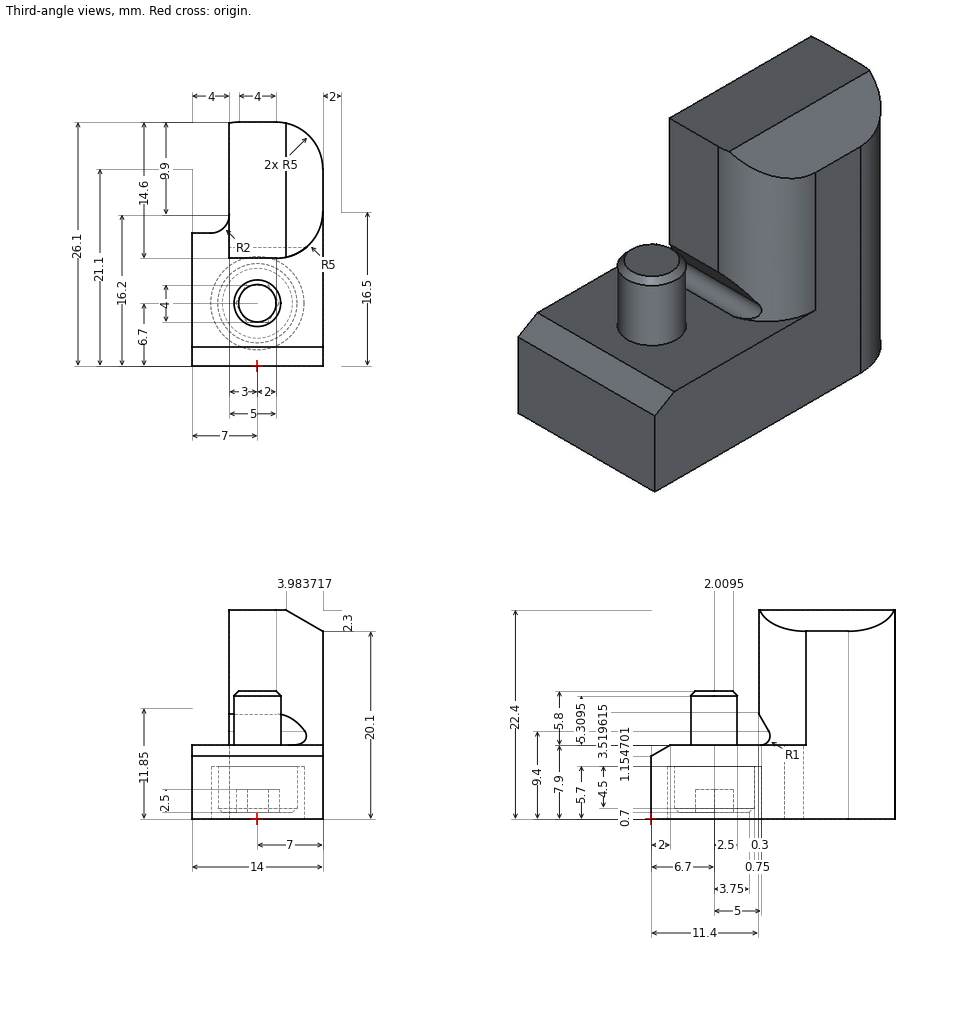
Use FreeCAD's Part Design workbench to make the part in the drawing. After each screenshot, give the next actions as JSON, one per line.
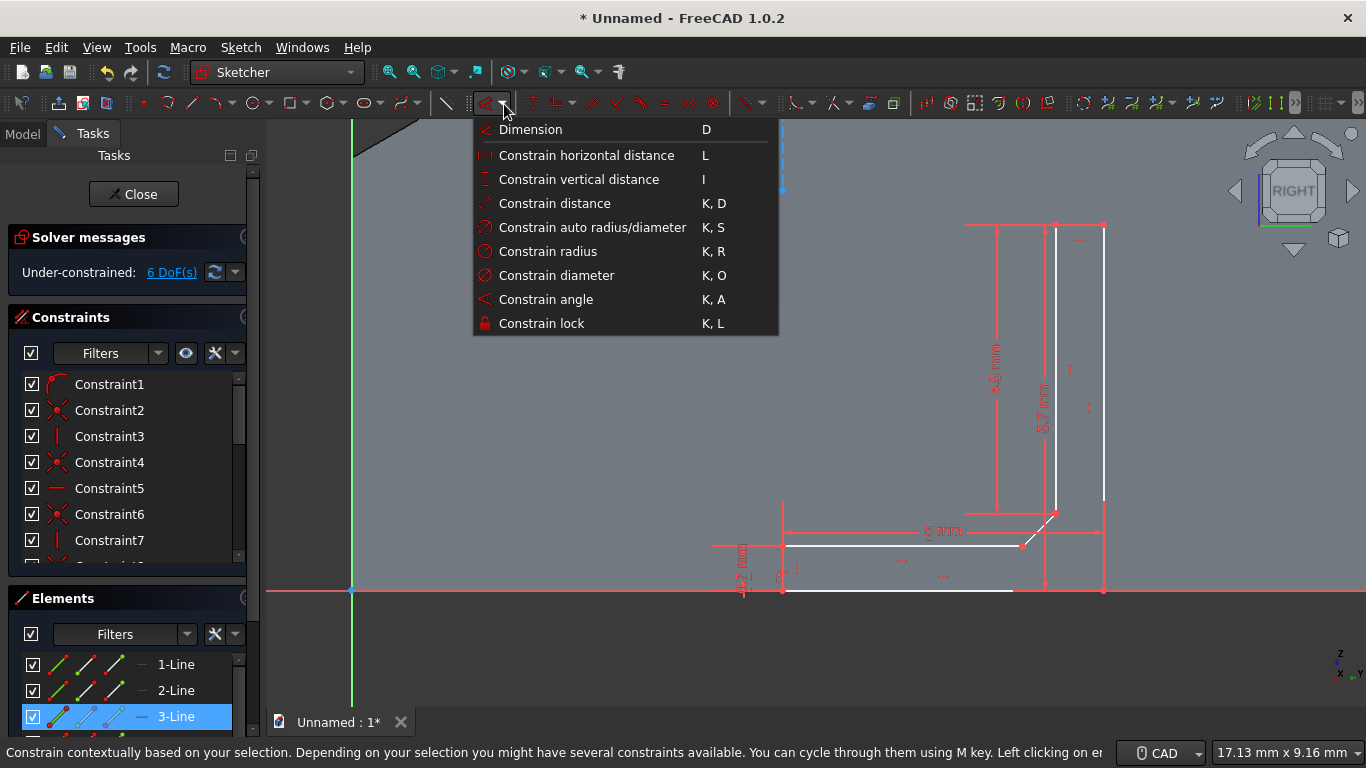
{"action": "left_click", "coordinate": [626, 155]}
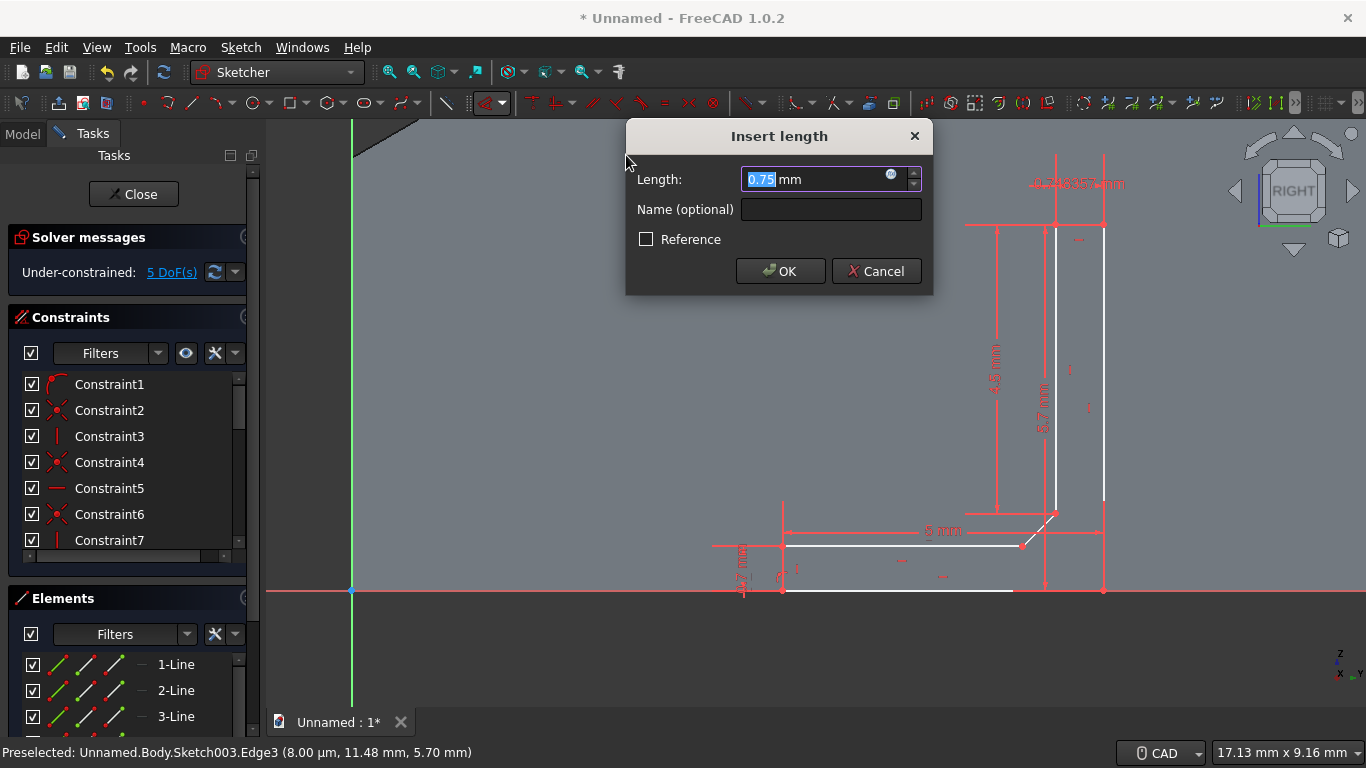
{"action": "type", "text": "0.75"}
{"action": "key", "text": "Return"}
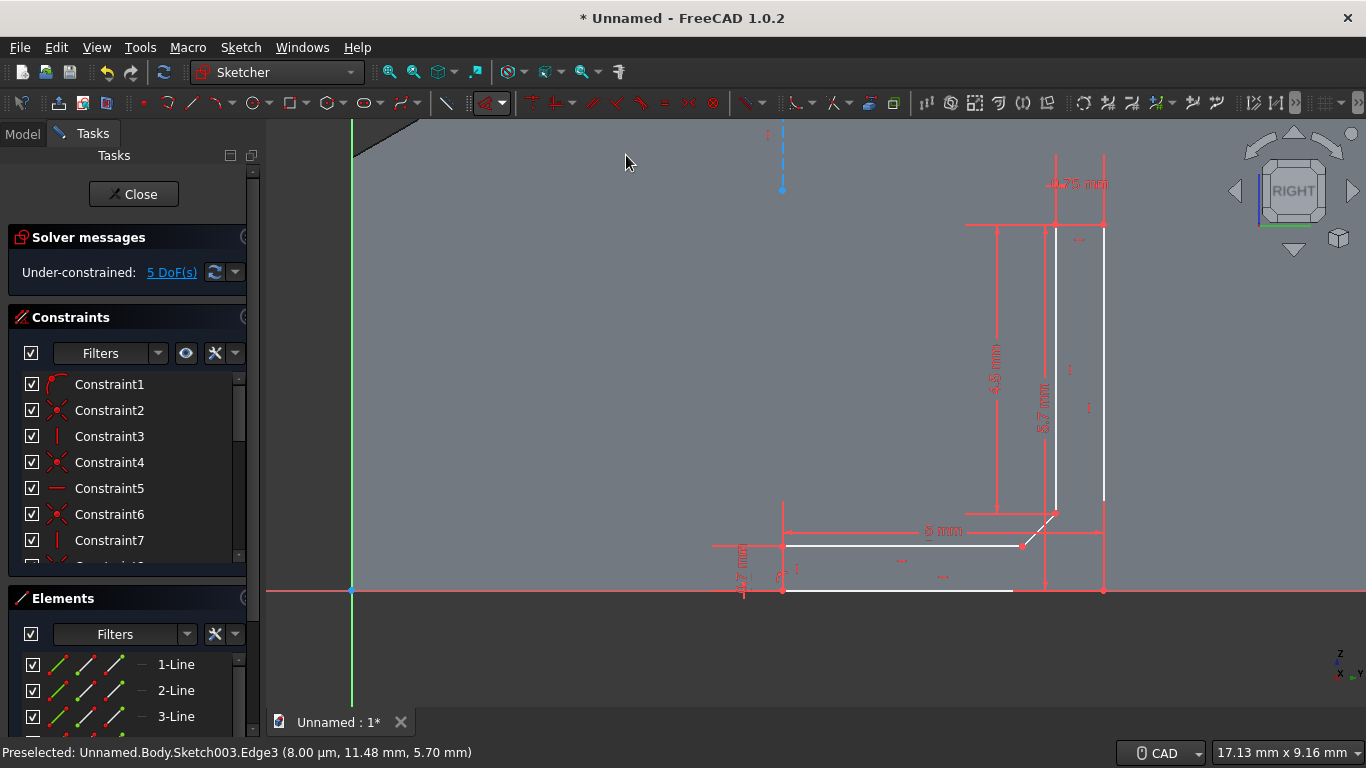
{"action": "left_click", "coordinate": [951, 546]}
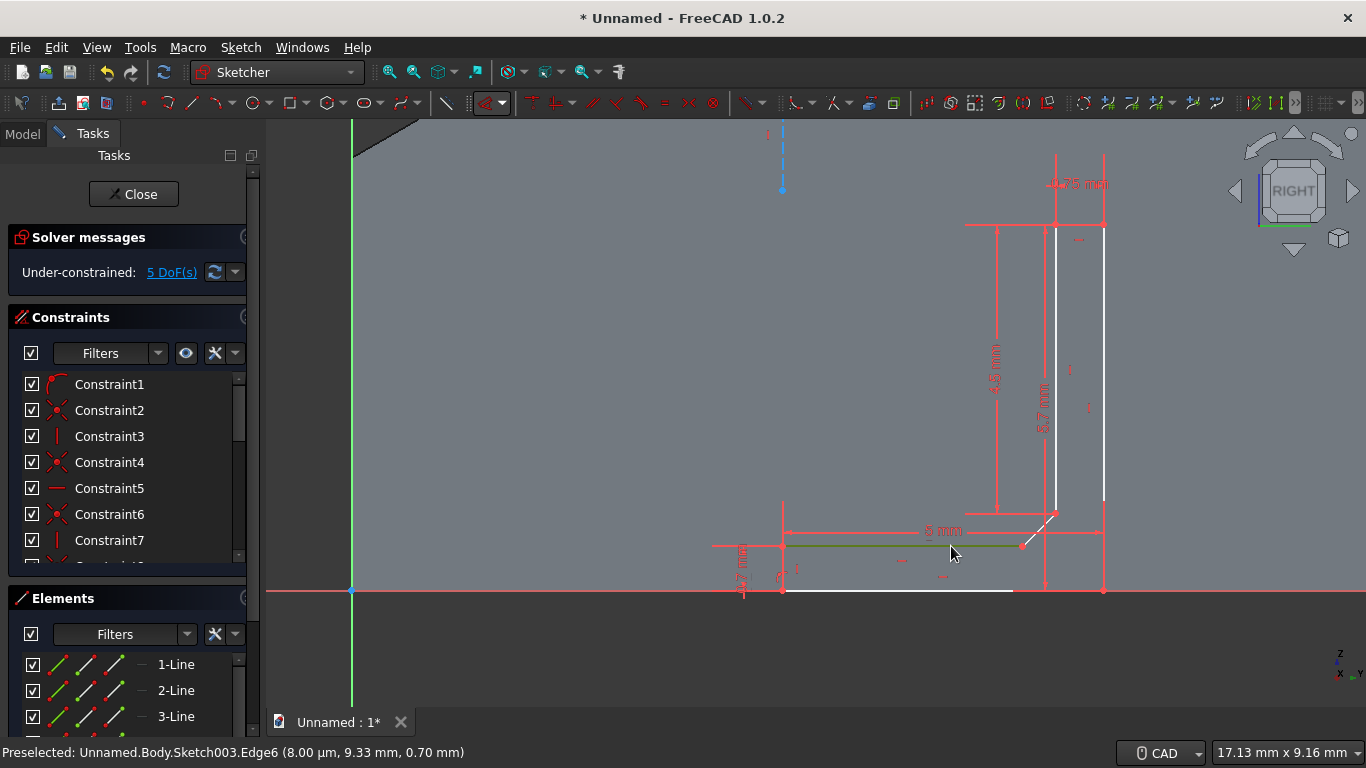
{"action": "key", "text": "l"}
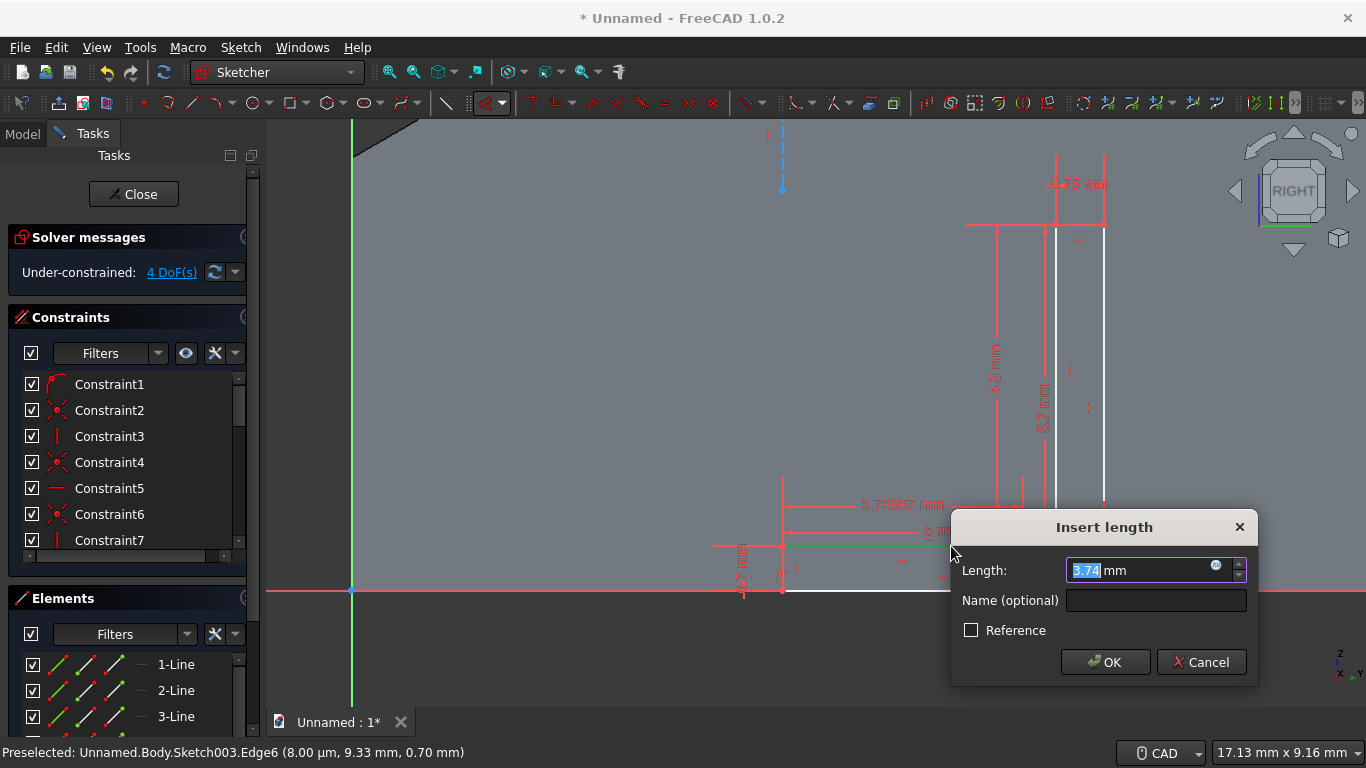
{"action": "type", "text": "3.75"}
{"action": "key", "text": "Return"}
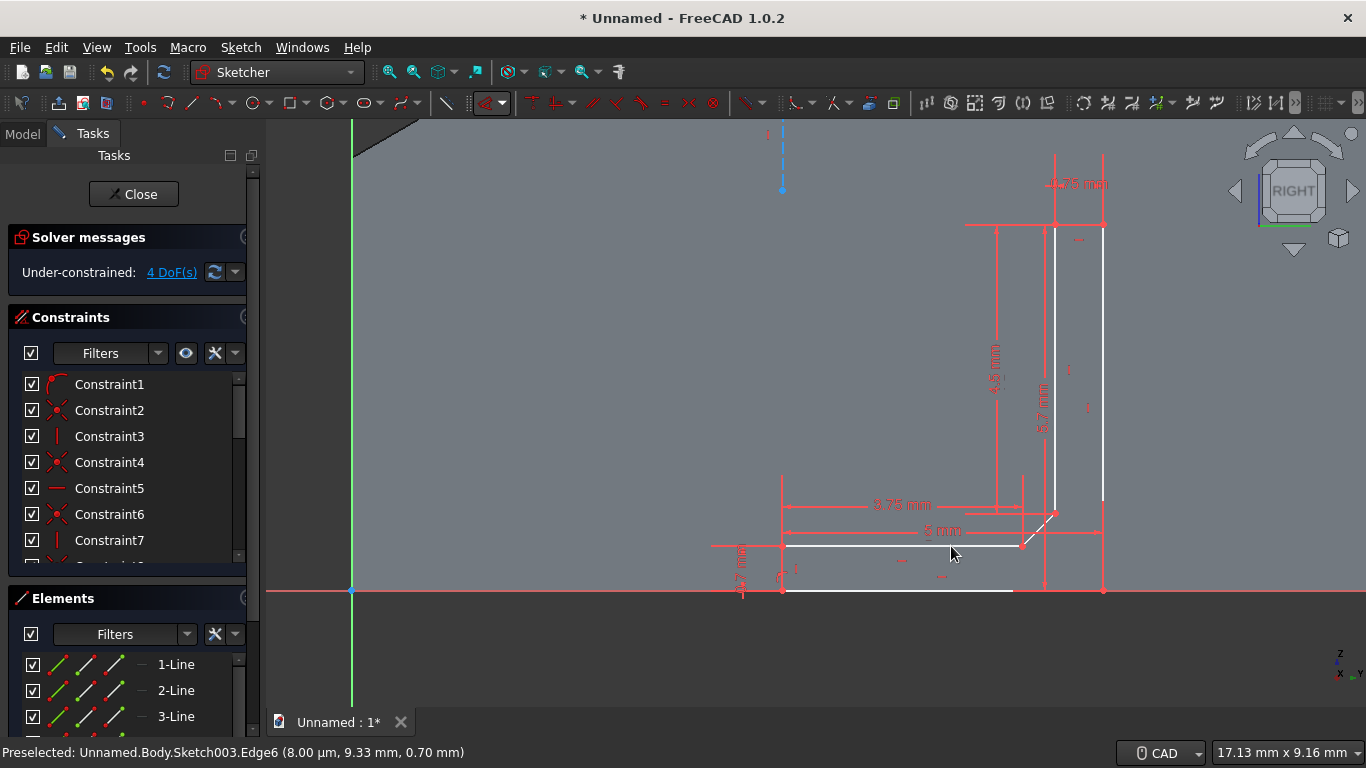
{"action": "left_click", "coordinate": [782, 591]}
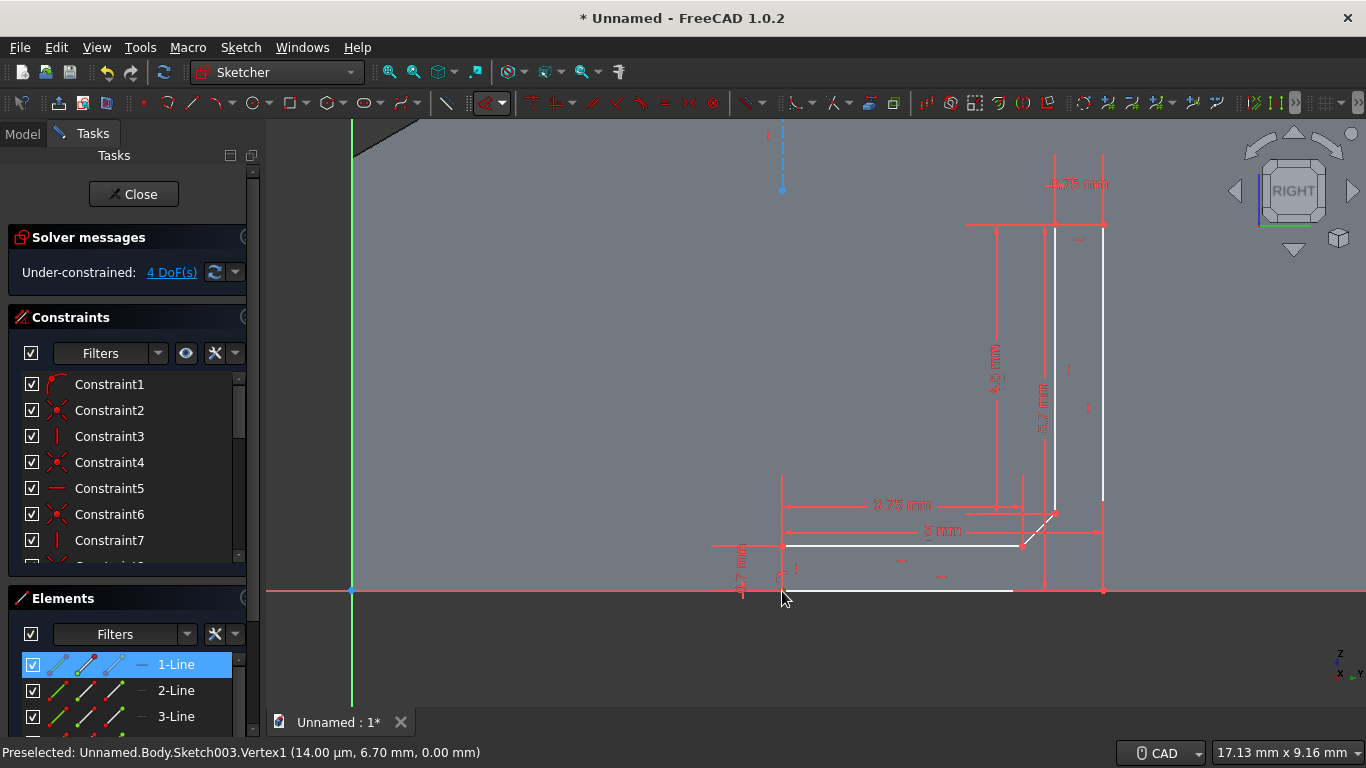
{"action": "left_click", "coordinate": [504, 104]}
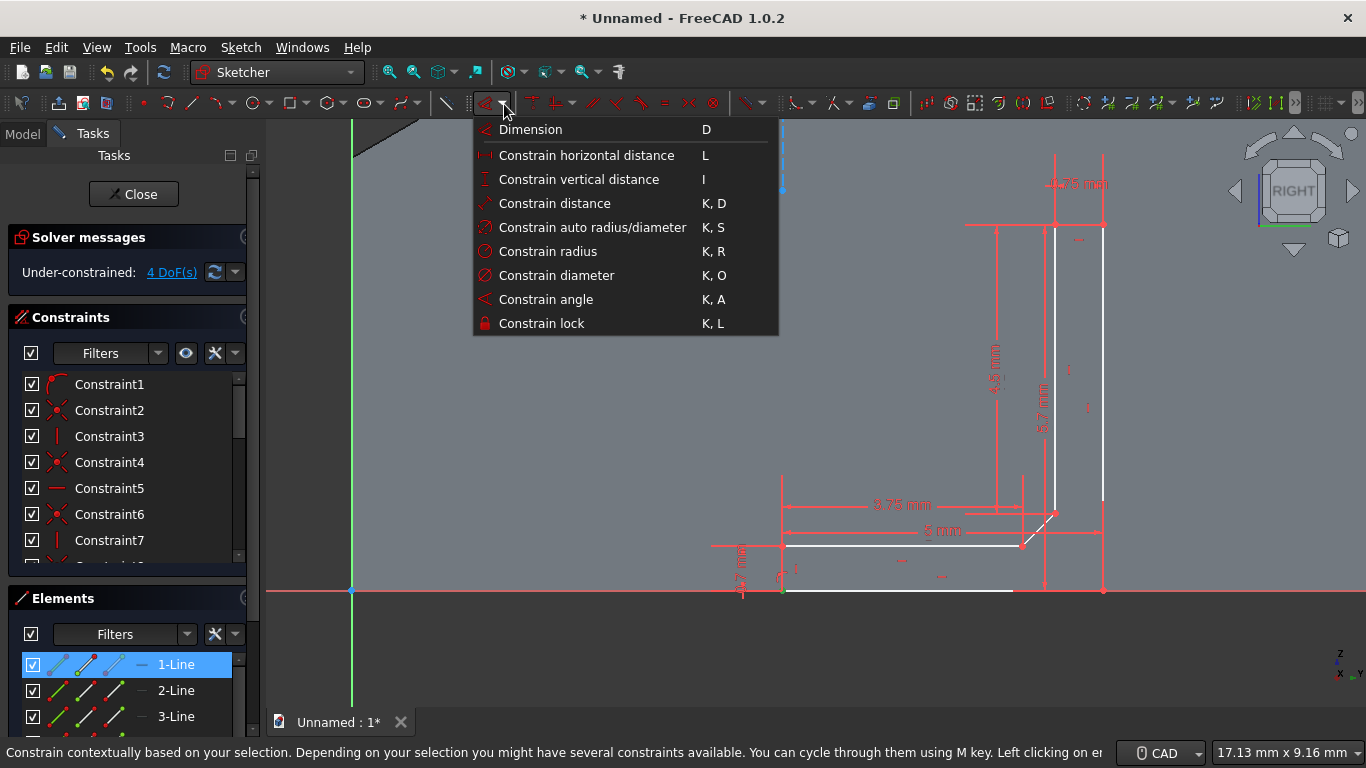
{"action": "left_click", "coordinate": [626, 155]}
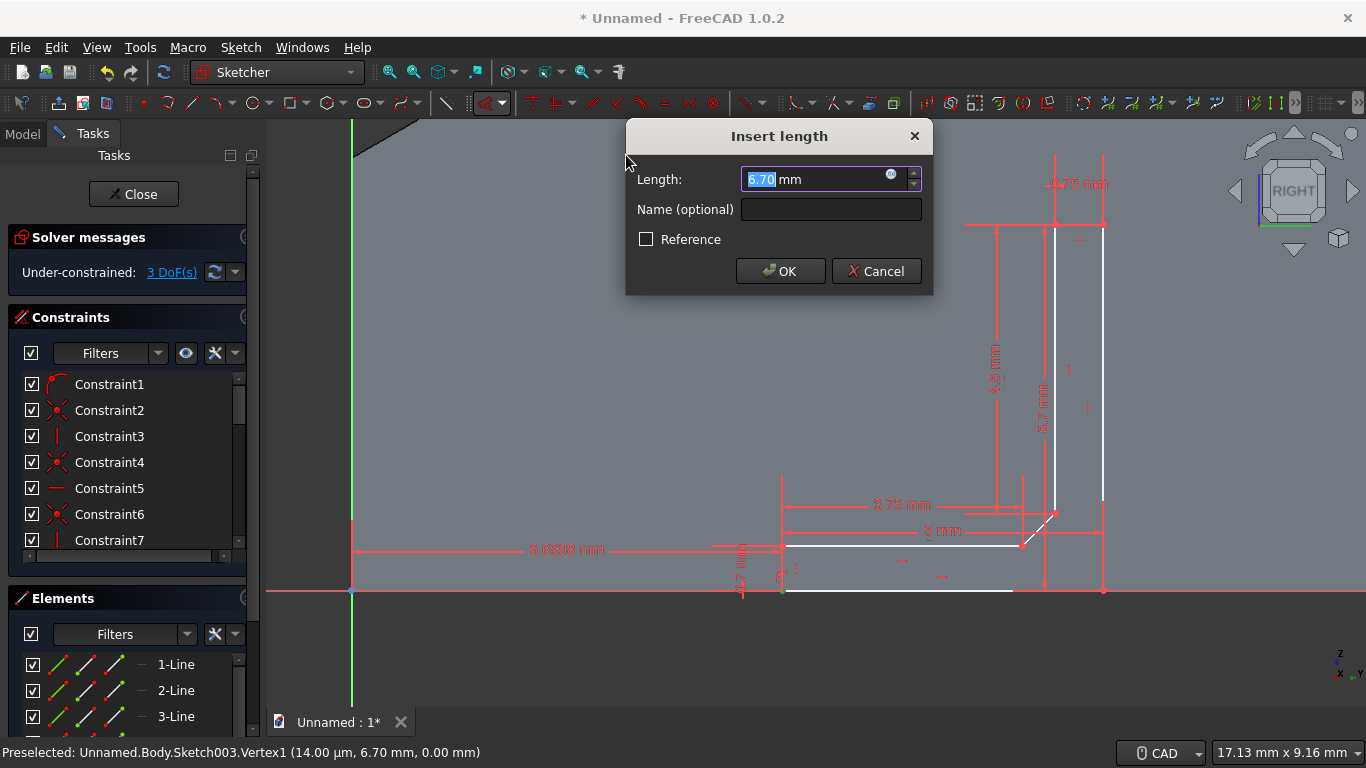
{"action": "type", "text": "6.7"}
{"action": "key", "text": "Return"}